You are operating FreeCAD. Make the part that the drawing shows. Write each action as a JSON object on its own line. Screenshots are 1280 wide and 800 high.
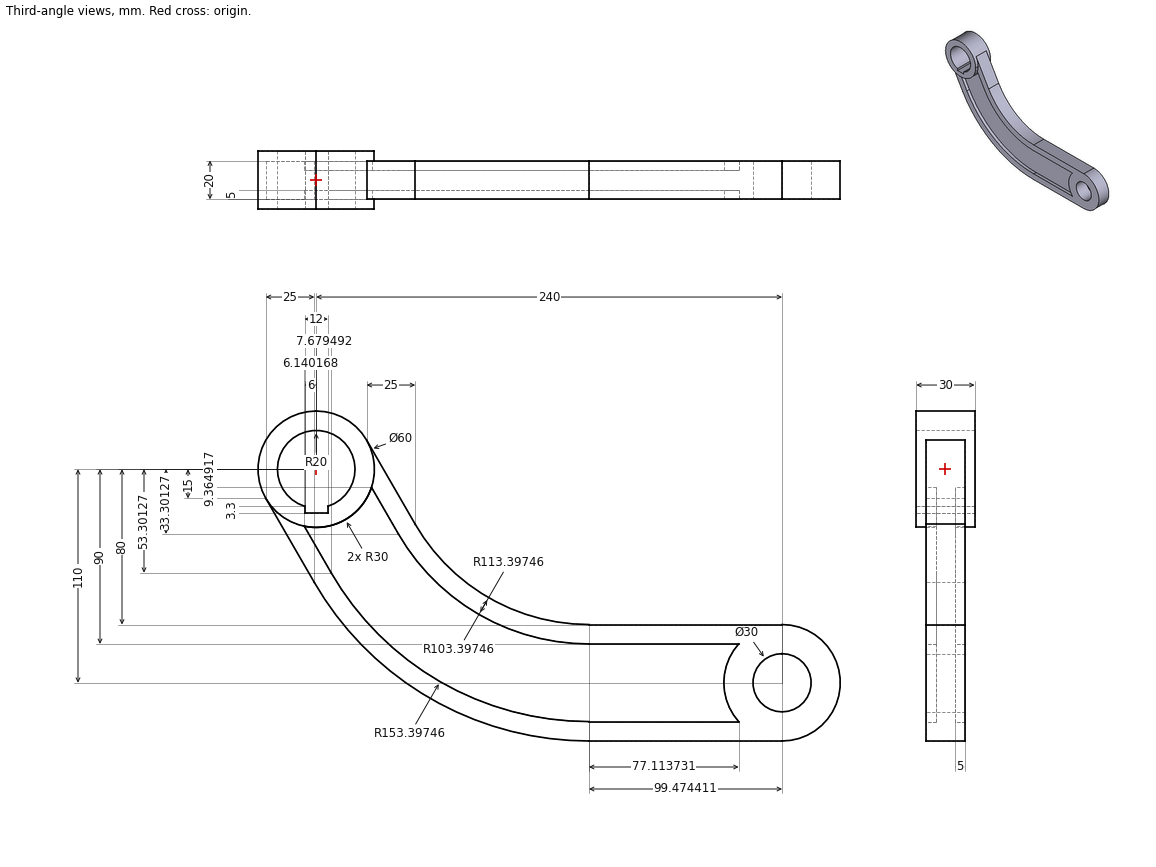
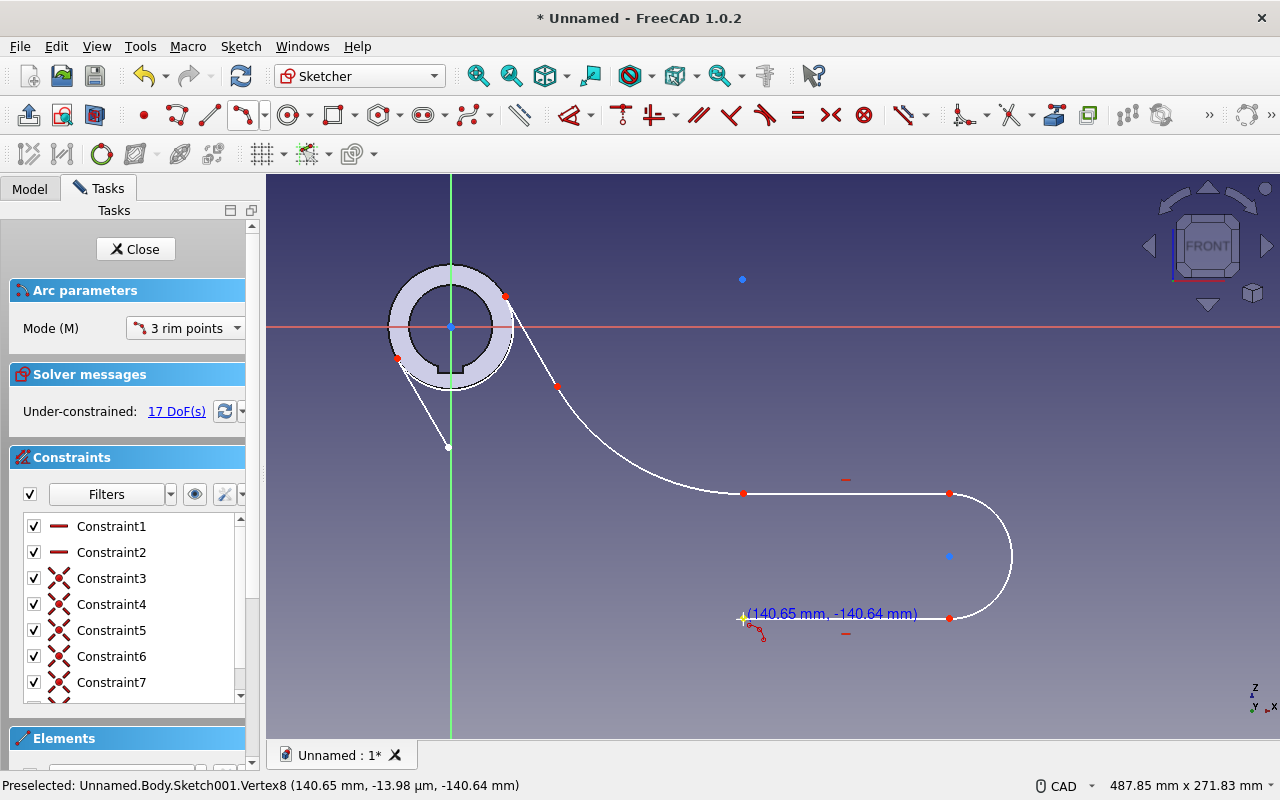
{"action": "scroll", "coordinate": [449, 448], "scroll_direction": "up", "scroll_amount": 11}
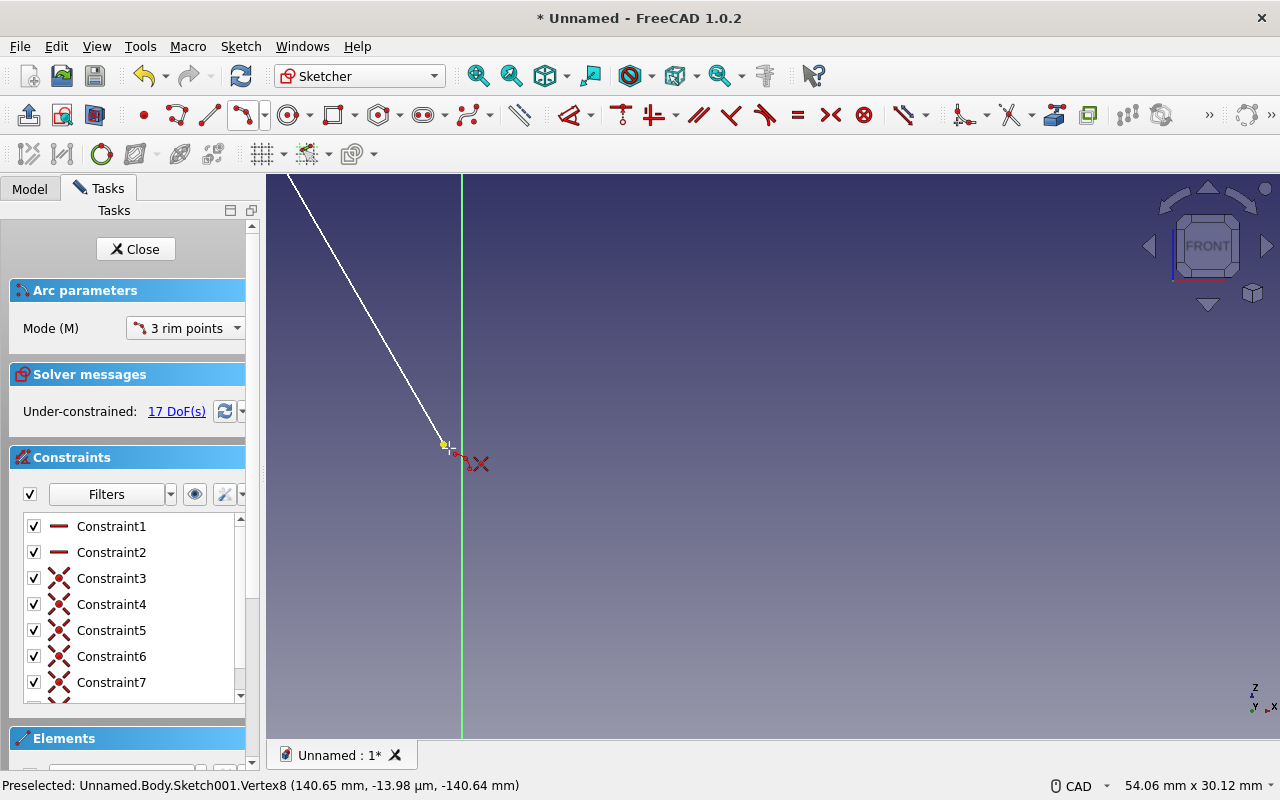
{"action": "left_click", "coordinate": [444, 444]}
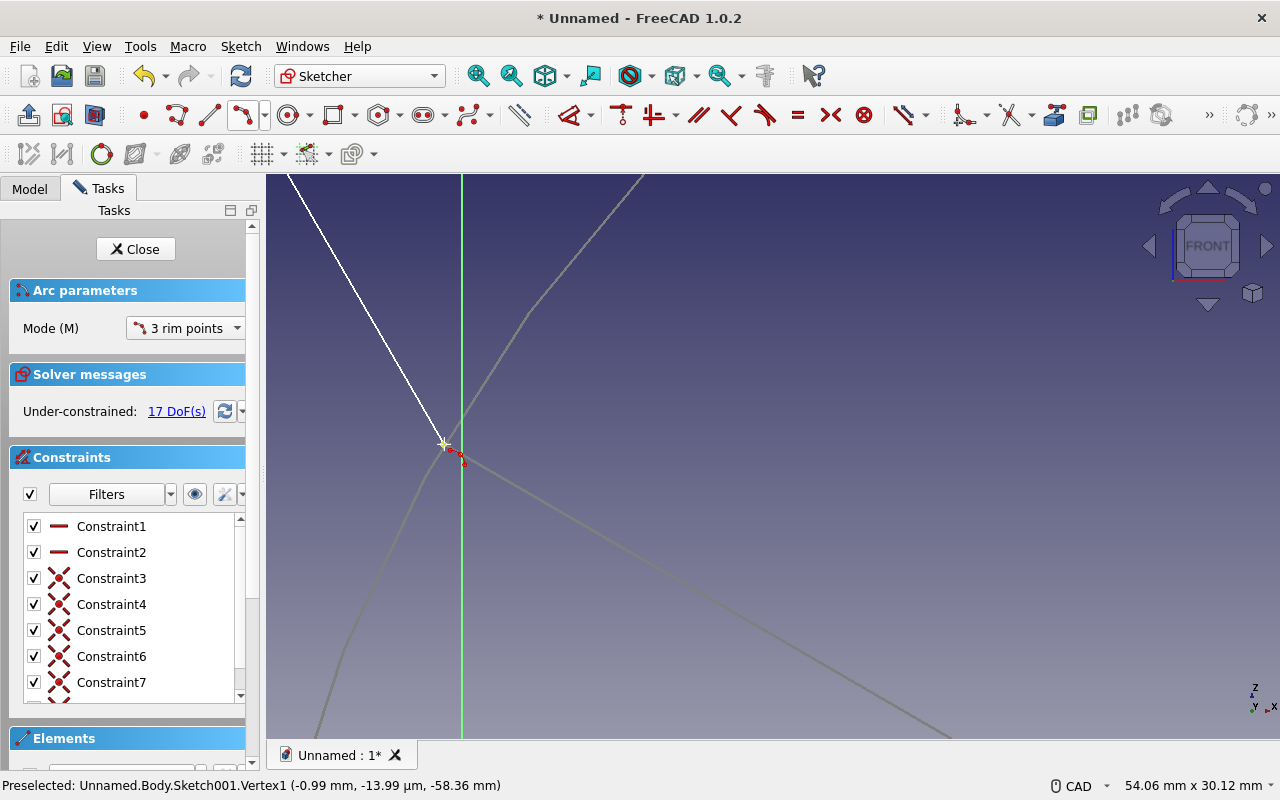
{"action": "scroll", "coordinate": [449, 448], "scroll_direction": "down", "scroll_amount": 11}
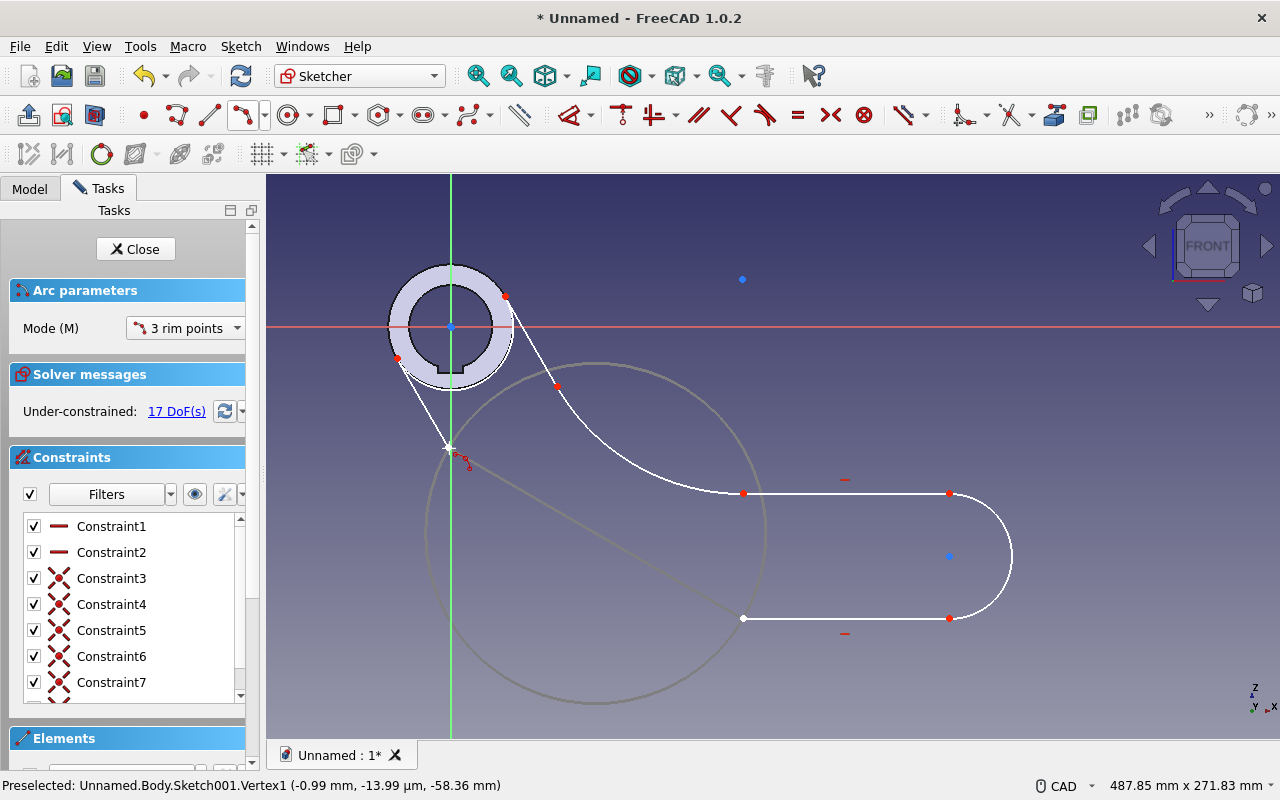
{"action": "left_click", "coordinate": [573, 572]}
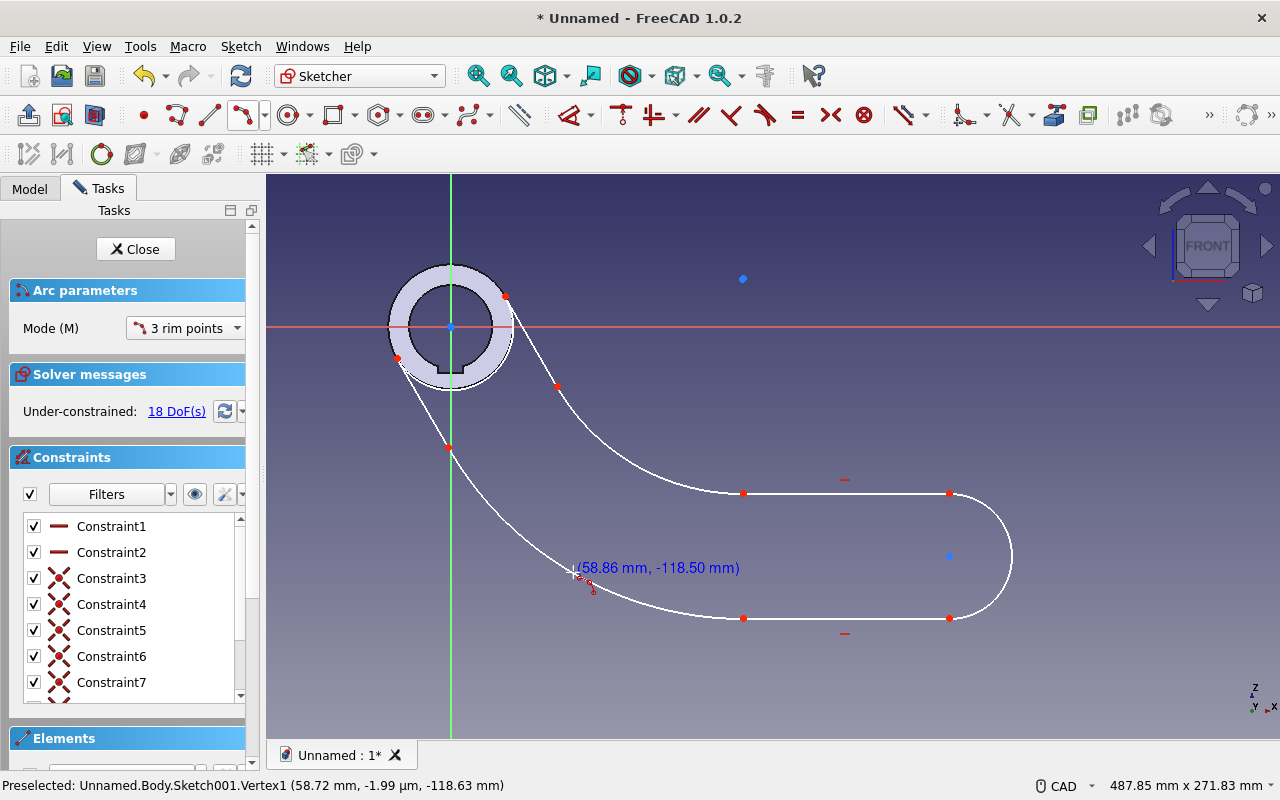
{"action": "key", "text": "g c"}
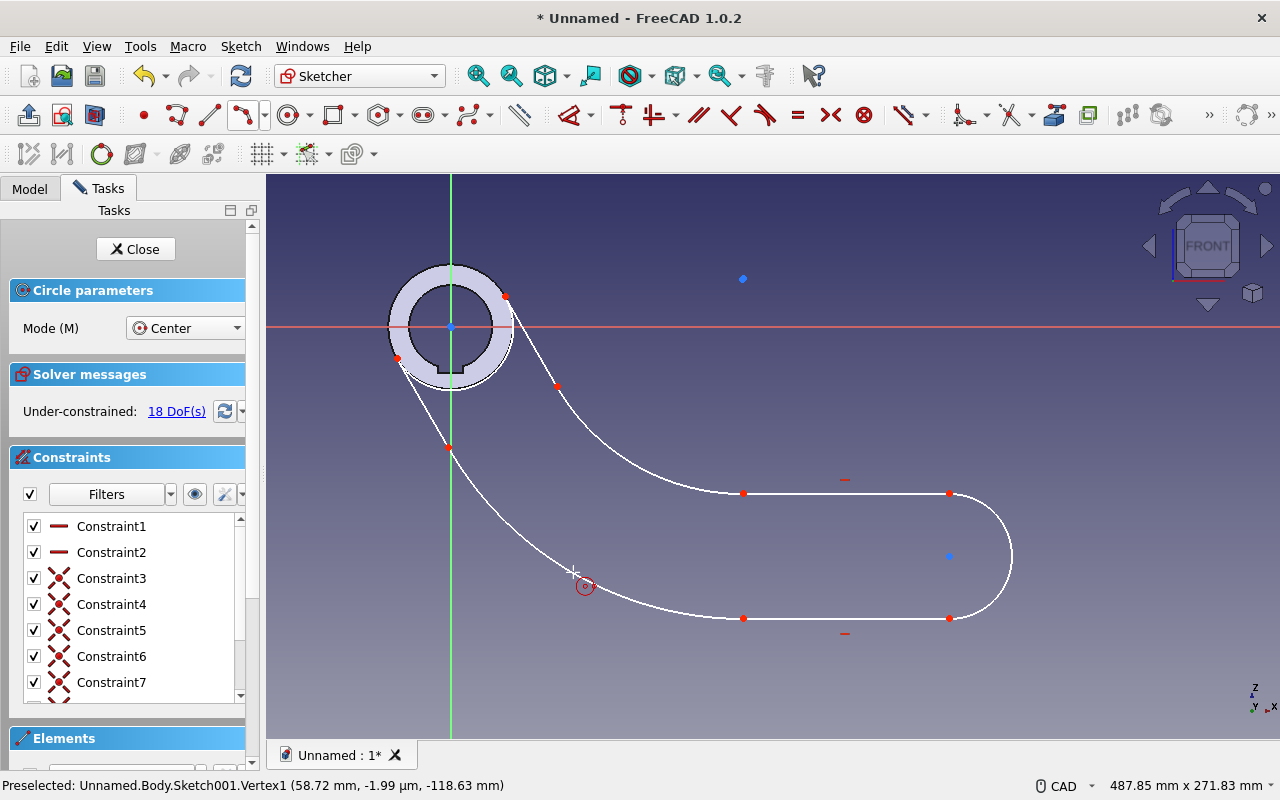
{"action": "left_click", "coordinate": [949, 555]}
{"action": "mouse_move", "coordinate": [972, 533]}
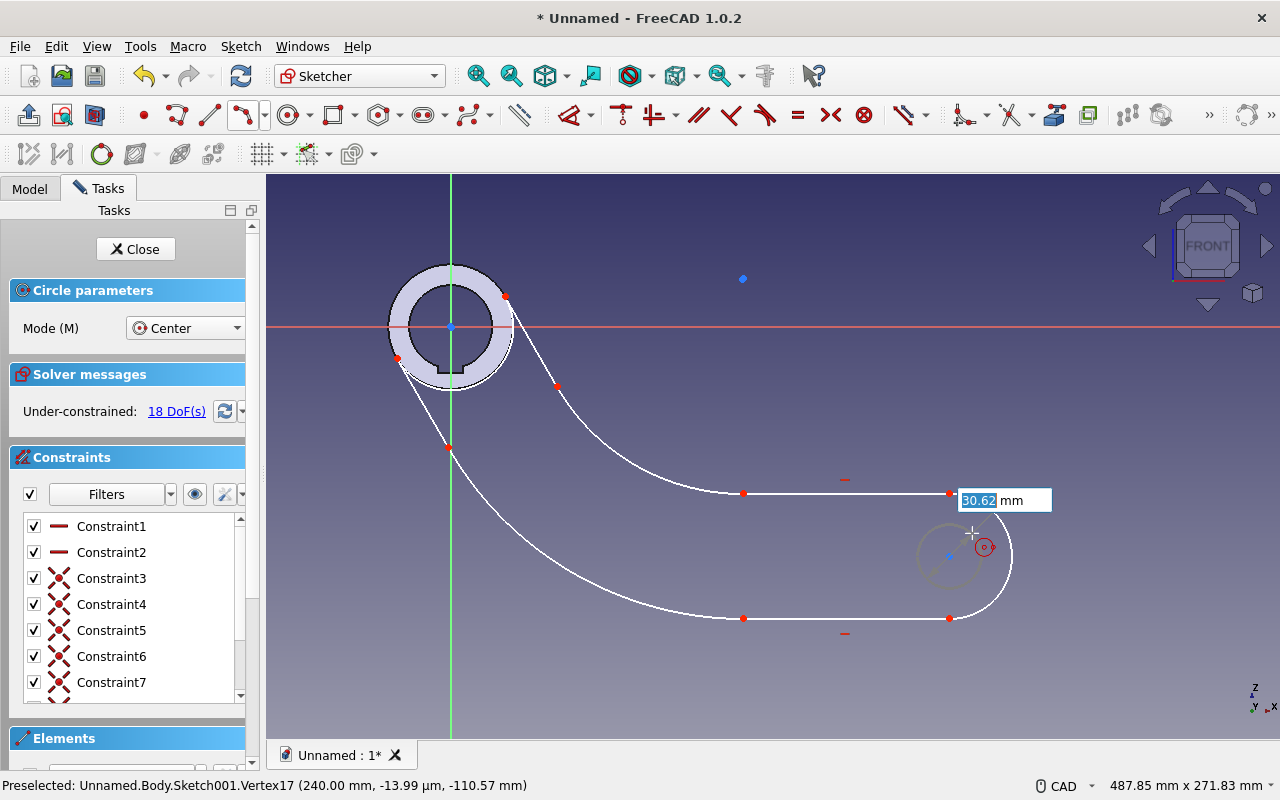
{"action": "type", "text": "30"}
{"action": "key", "text": "Return"}
{"action": "key", "text": "Escape"}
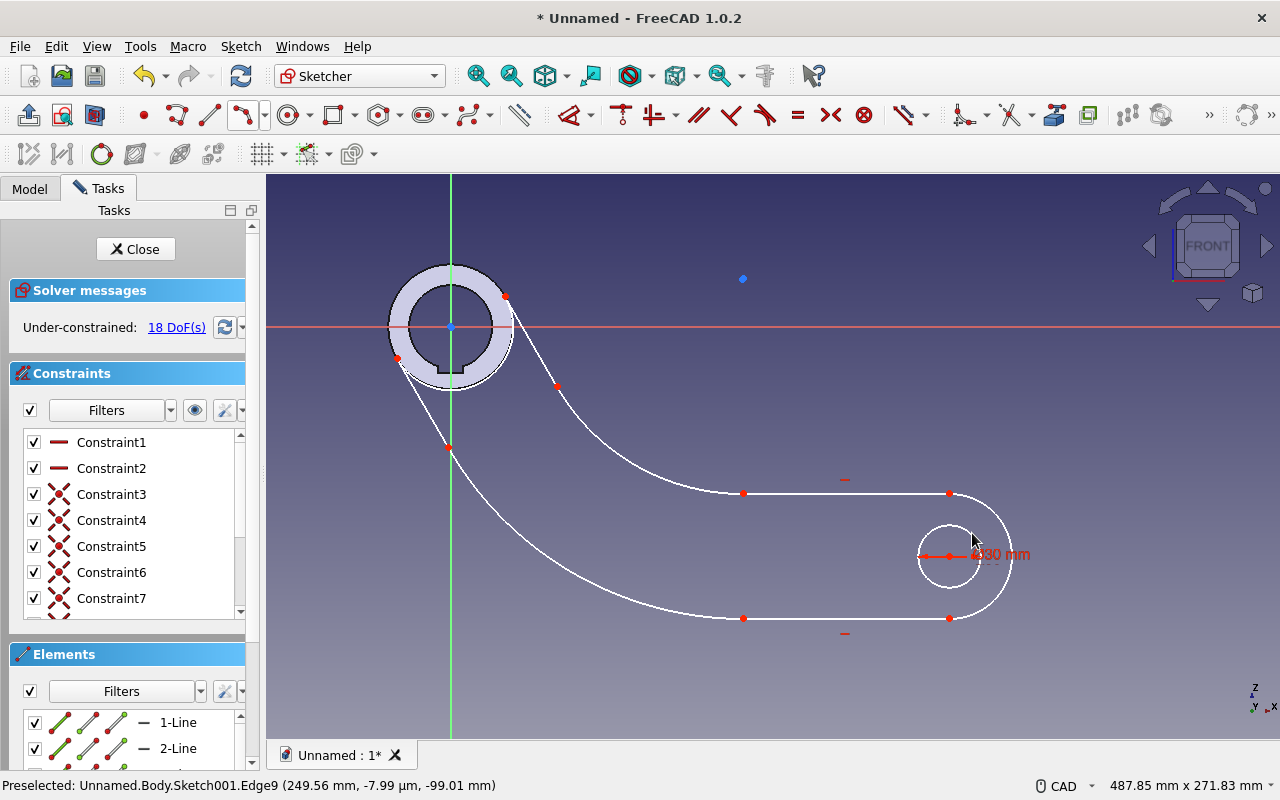
{"action": "left_click", "coordinate": [433, 421]}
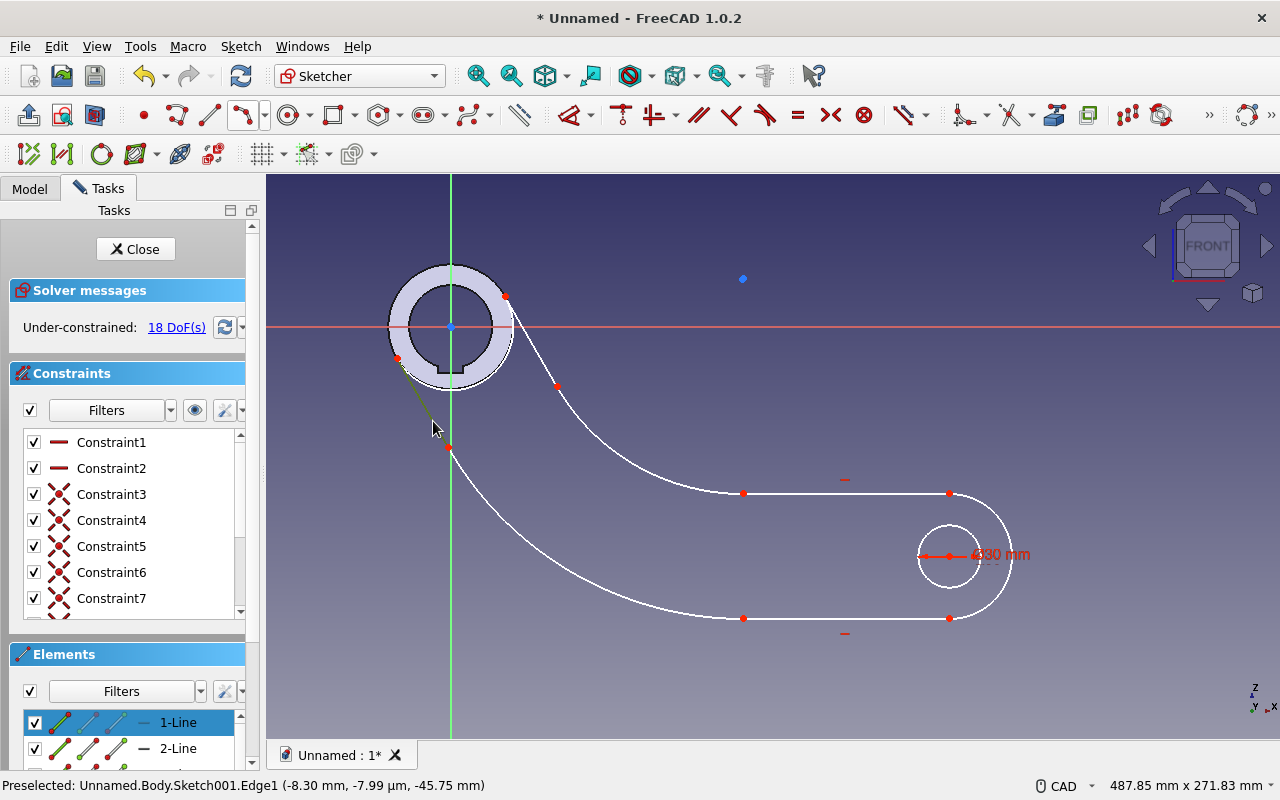
{"action": "left_click", "coordinate": [508, 353]}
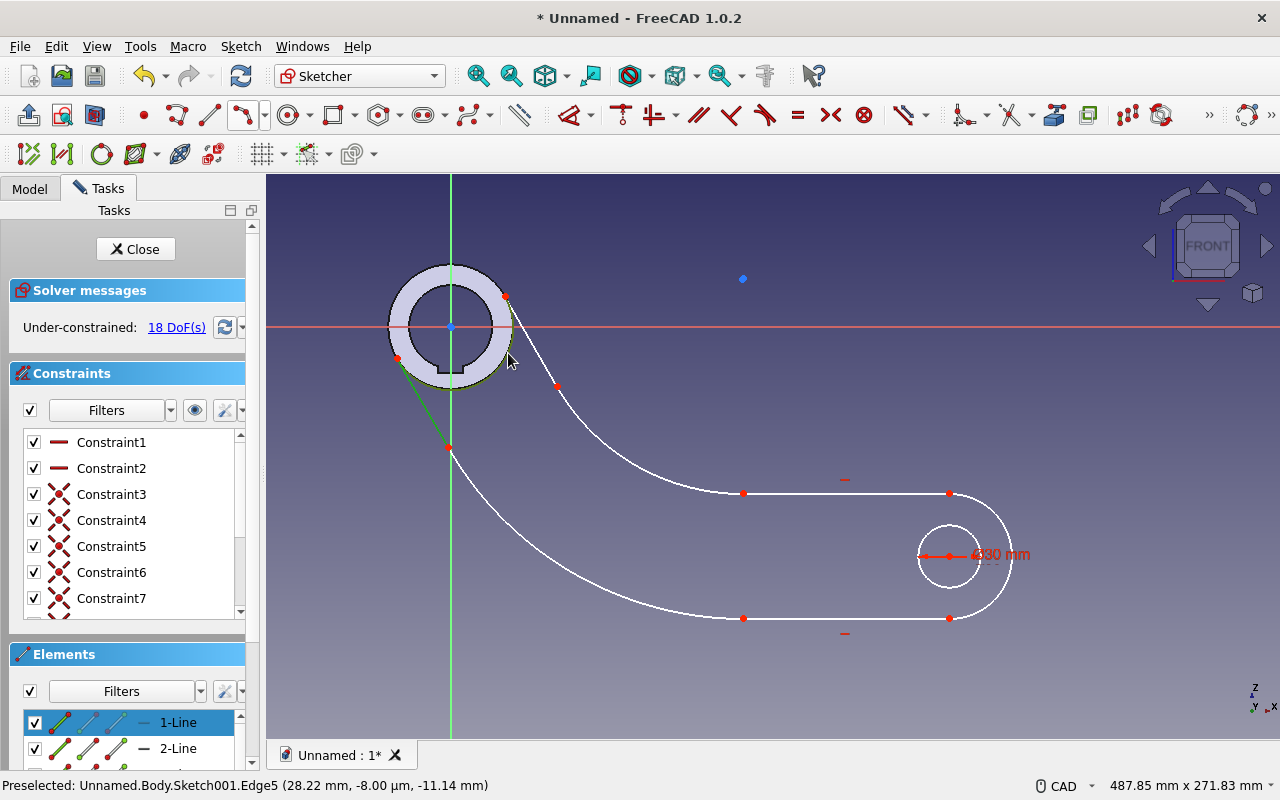
{"action": "left_click", "coordinate": [765, 116]}